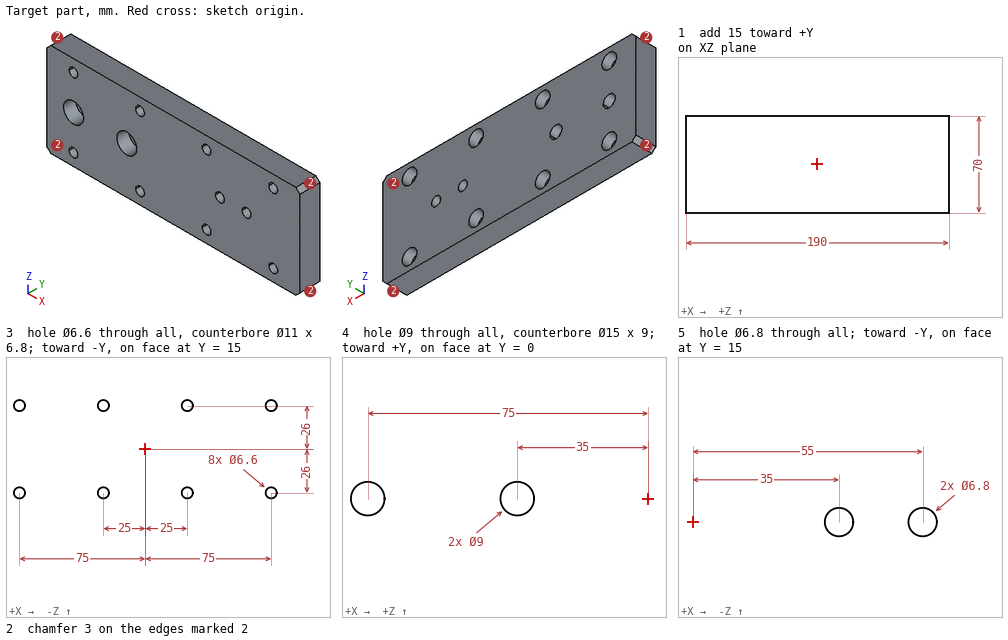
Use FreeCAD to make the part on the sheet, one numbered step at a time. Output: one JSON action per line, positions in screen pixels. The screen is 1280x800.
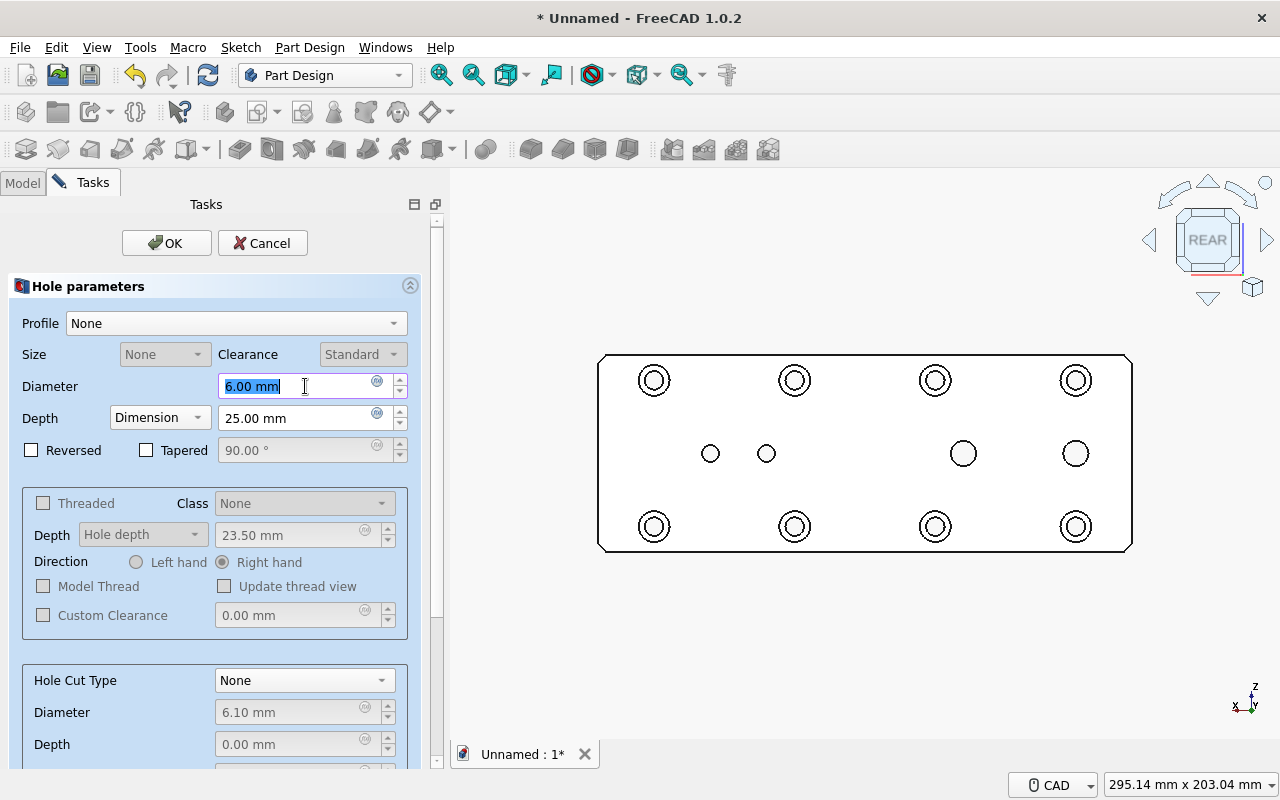
{"action": "type", "text": "6.8"}
{"action": "key", "text": "Tab"}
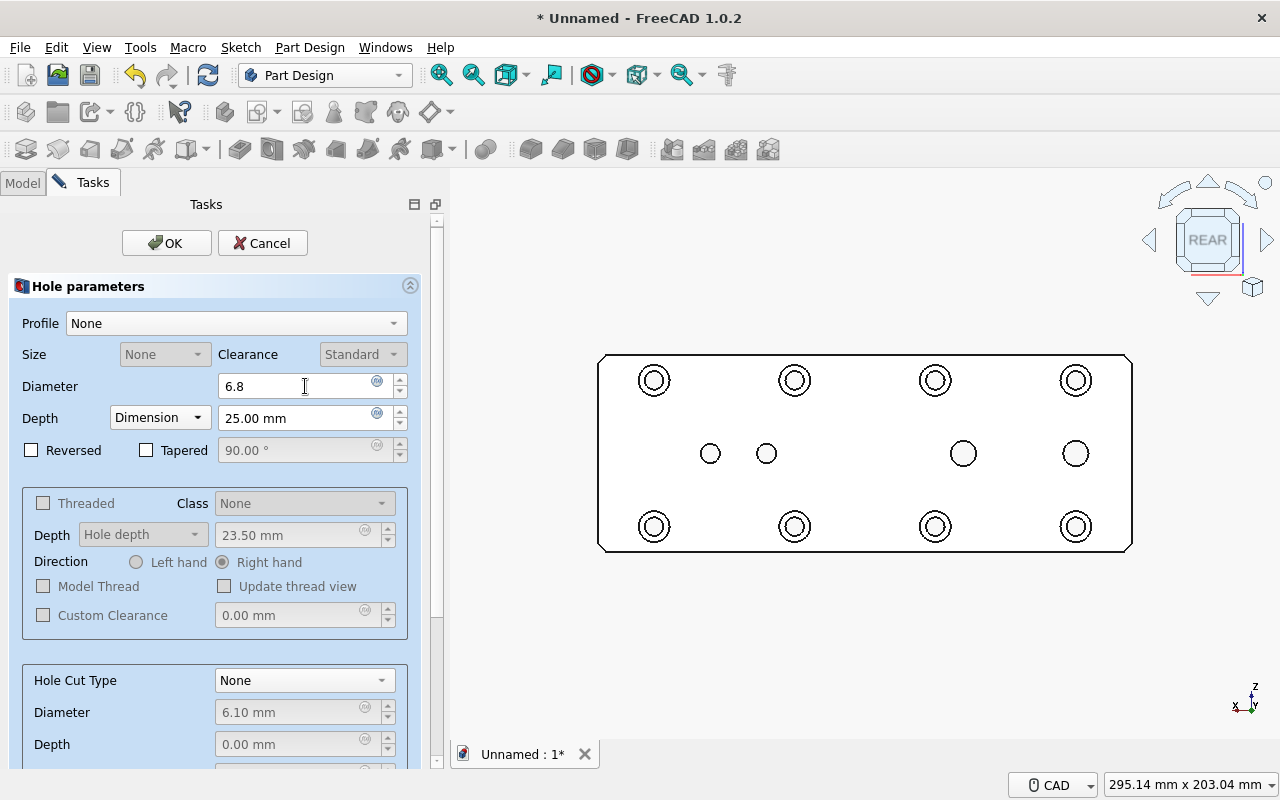
{"action": "left_click", "coordinate": [161, 418]}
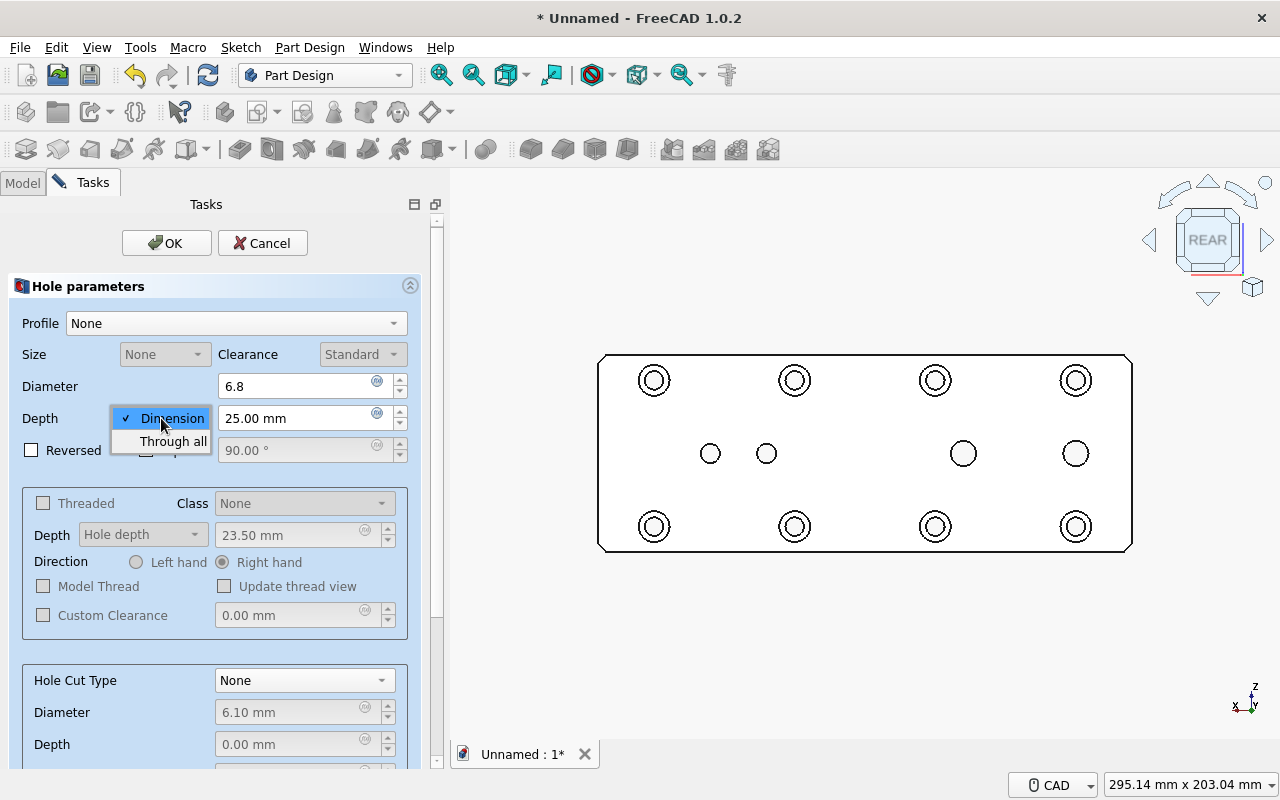
{"action": "left_click", "coordinate": [160, 442]}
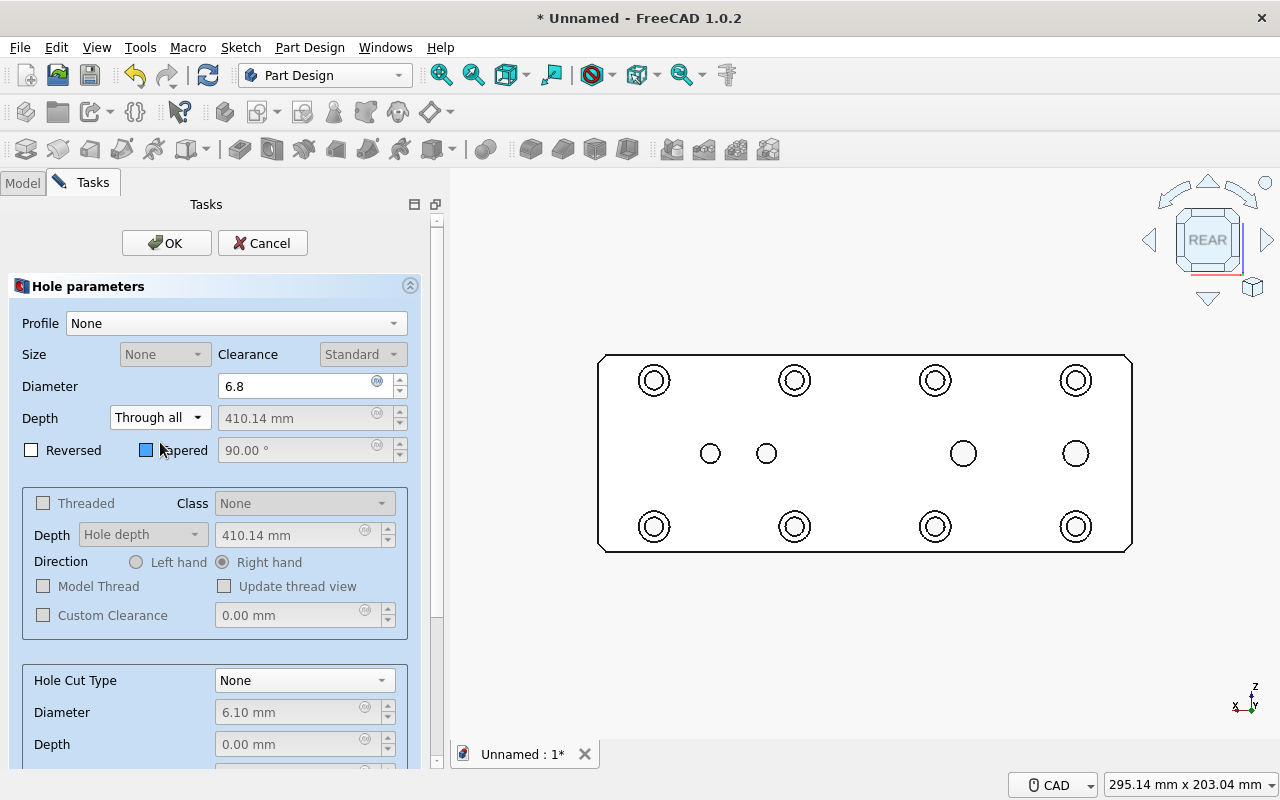
{"action": "left_click", "coordinate": [167, 243]}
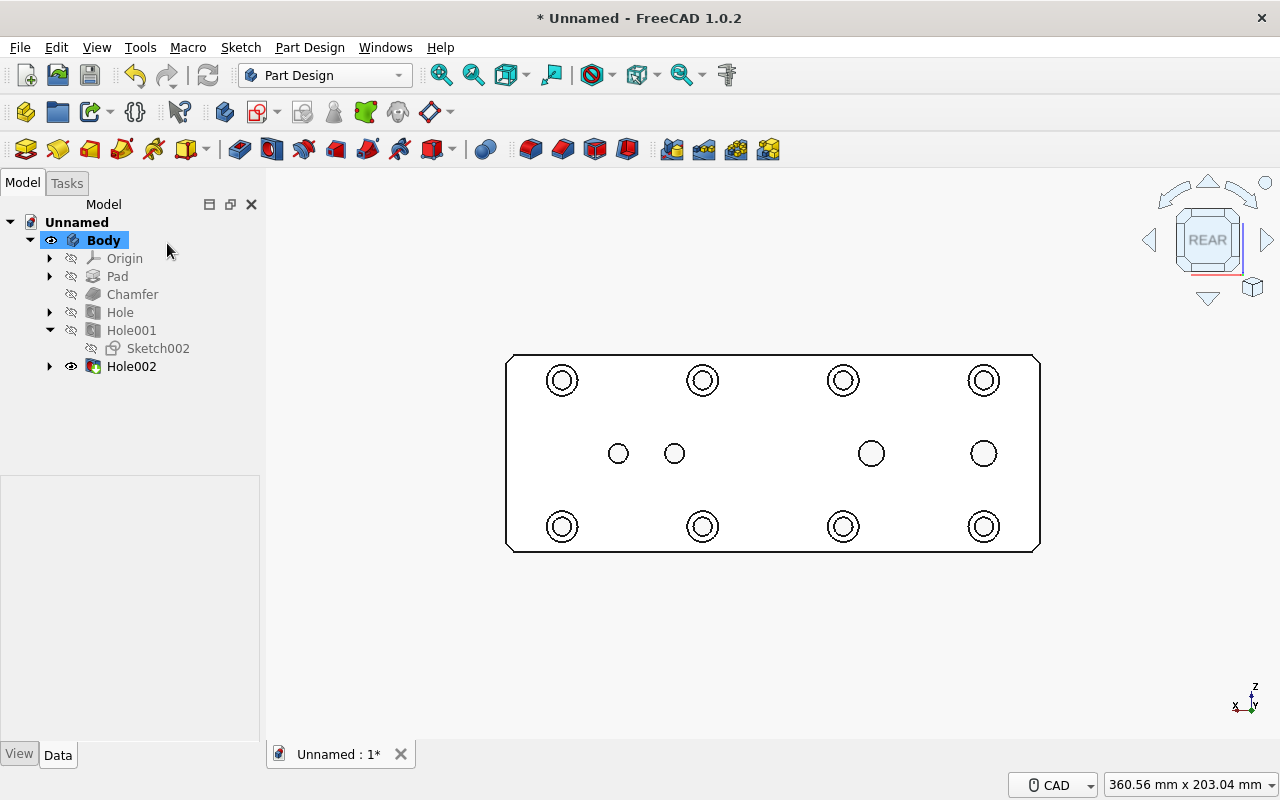
{"action": "key", "text": "0"}